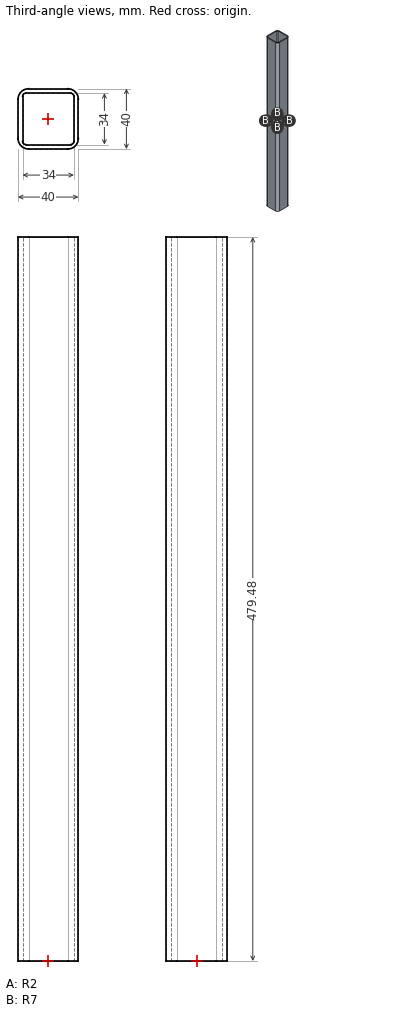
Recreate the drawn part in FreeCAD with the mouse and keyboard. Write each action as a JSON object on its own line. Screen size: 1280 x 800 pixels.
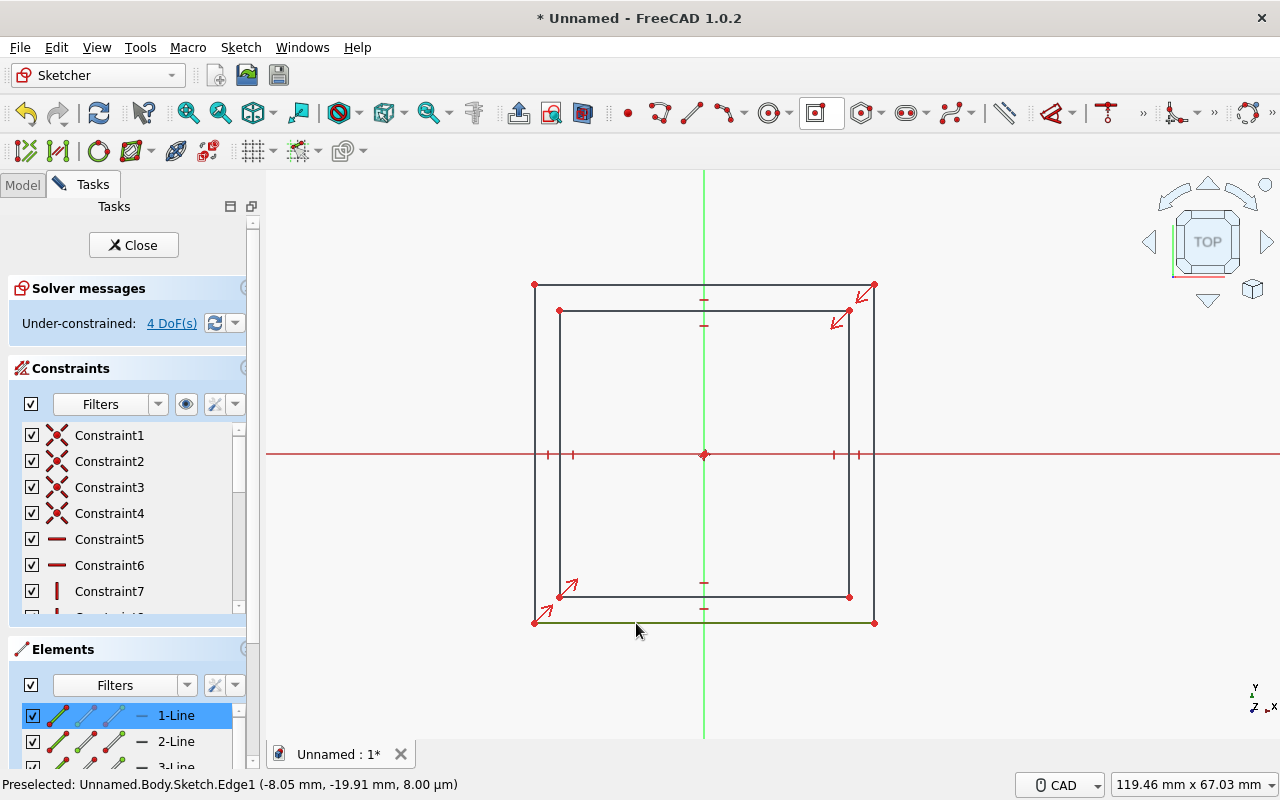
{"action": "left_click", "coordinate": [1074, 114]}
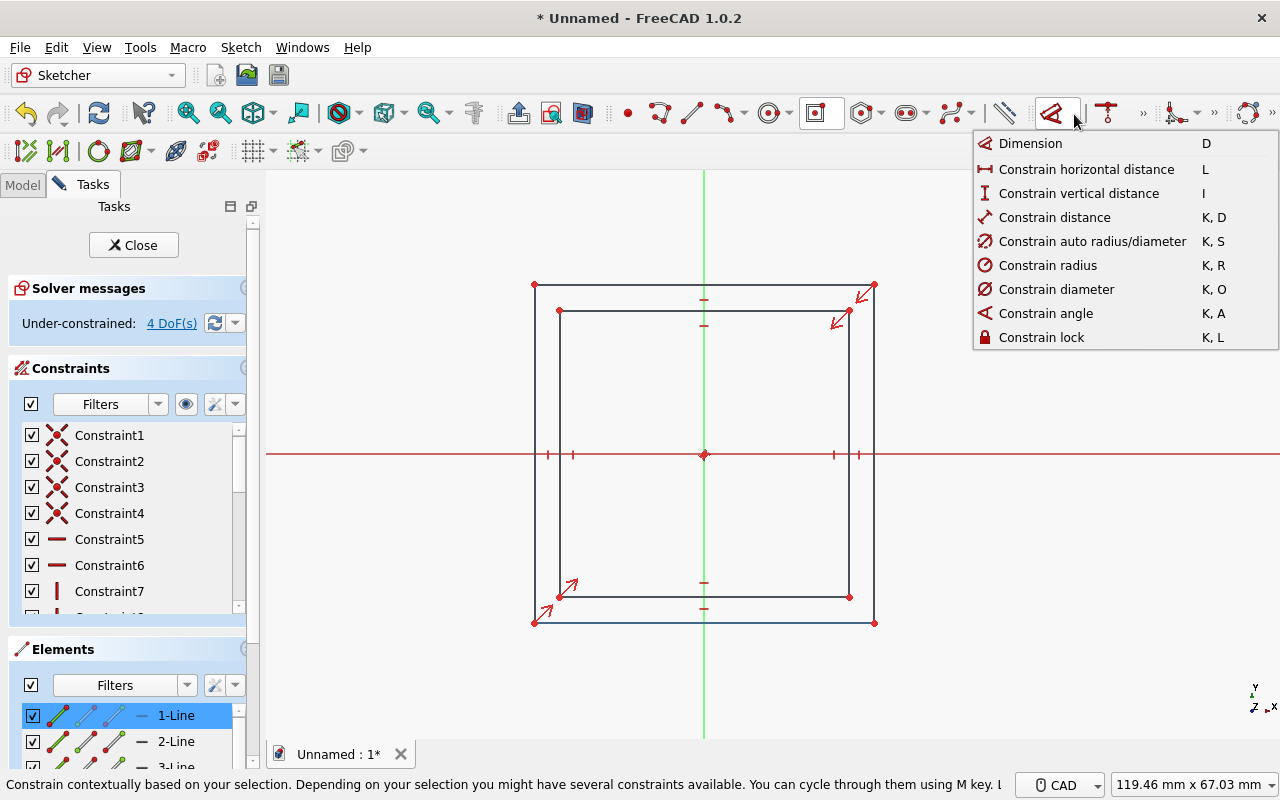
{"action": "left_click", "coordinate": [1126, 169]}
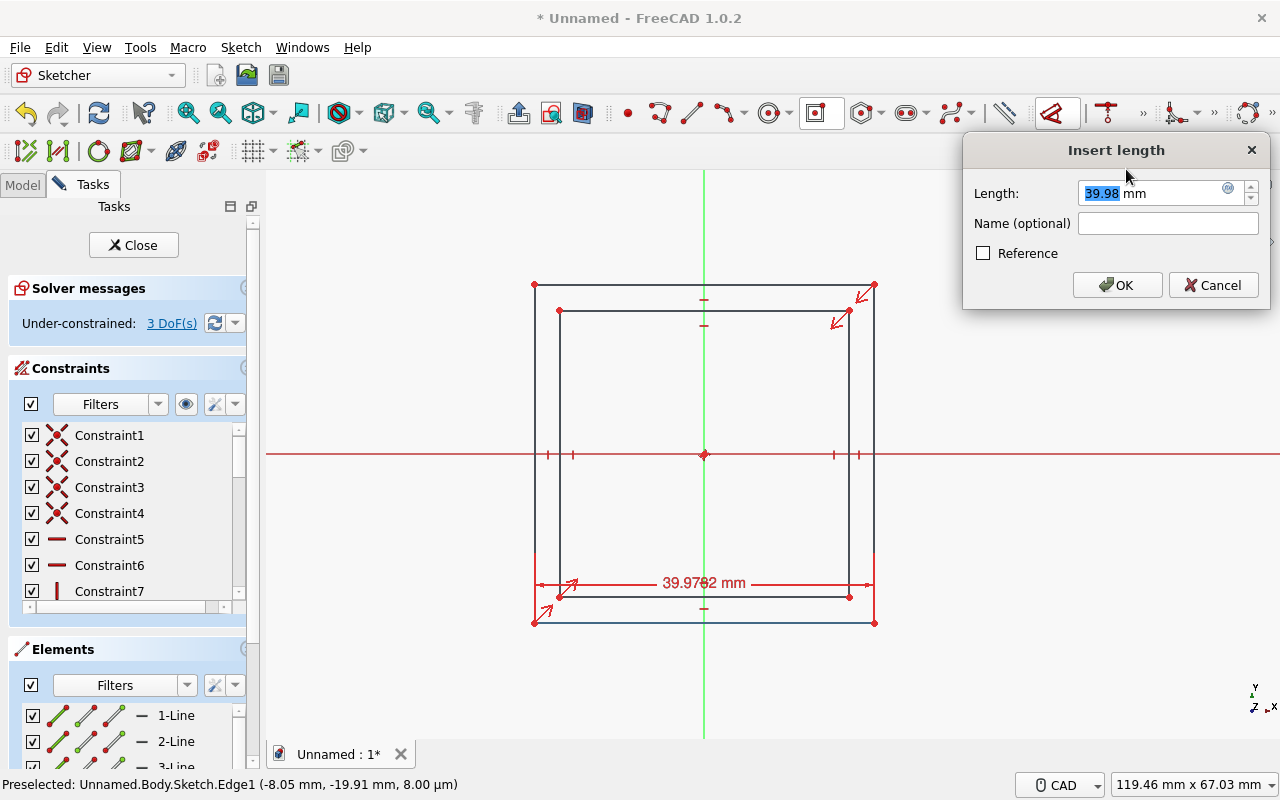
{"action": "type", "text": "40"}
{"action": "key", "text": "Return"}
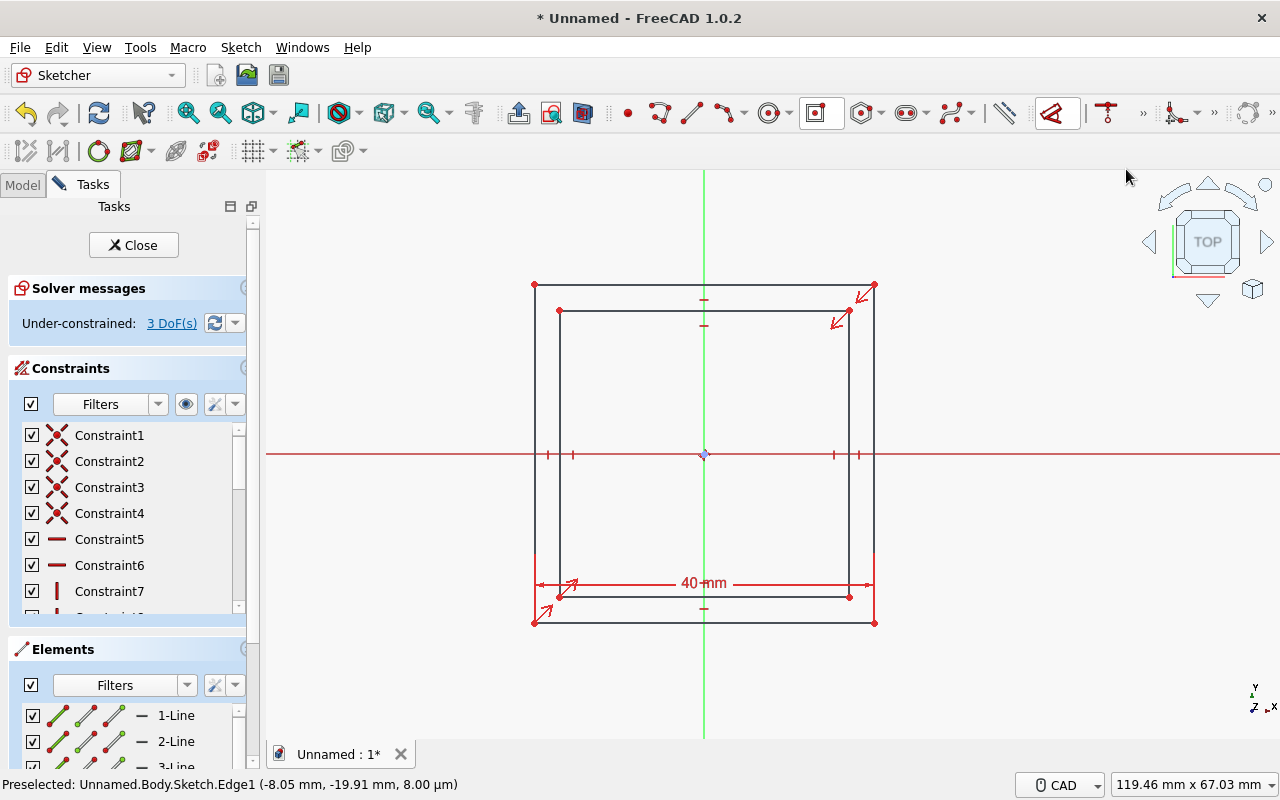
{"action": "left_click", "coordinate": [874, 522]}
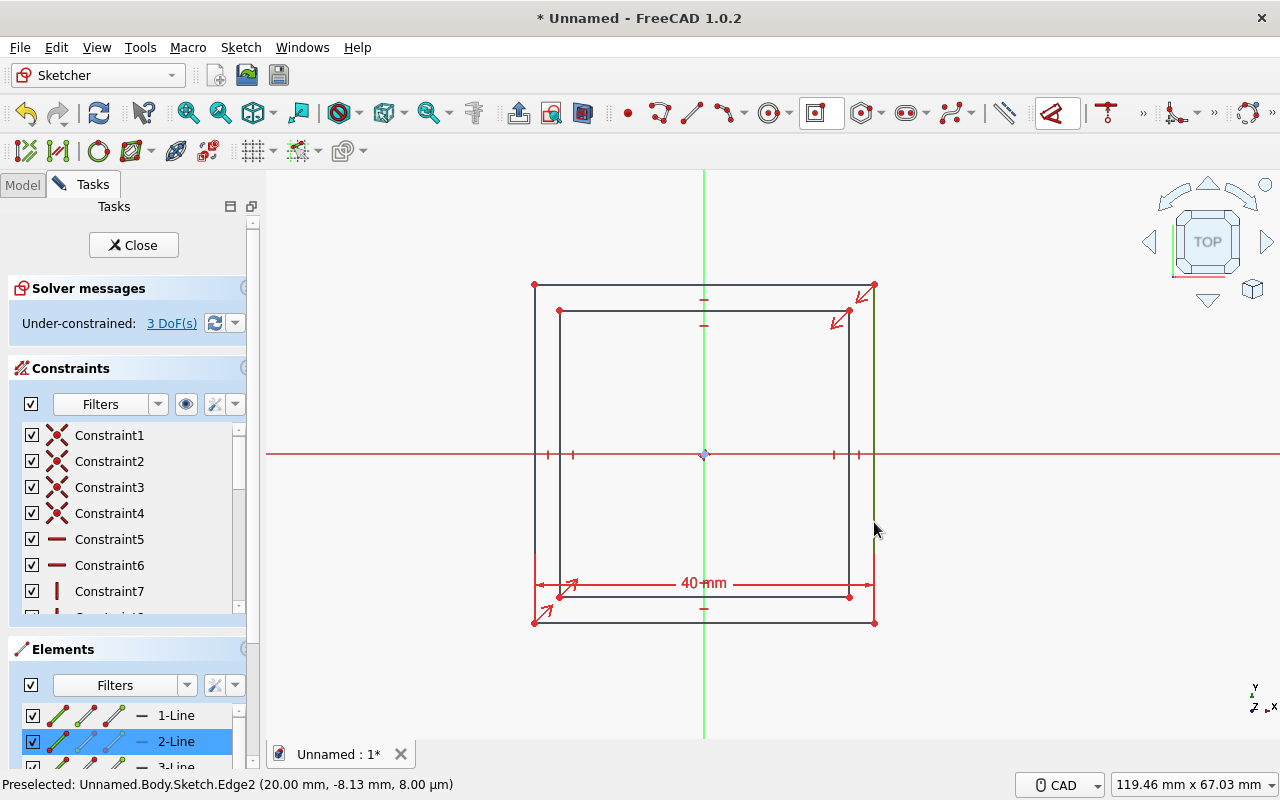
{"action": "key", "text": "i"}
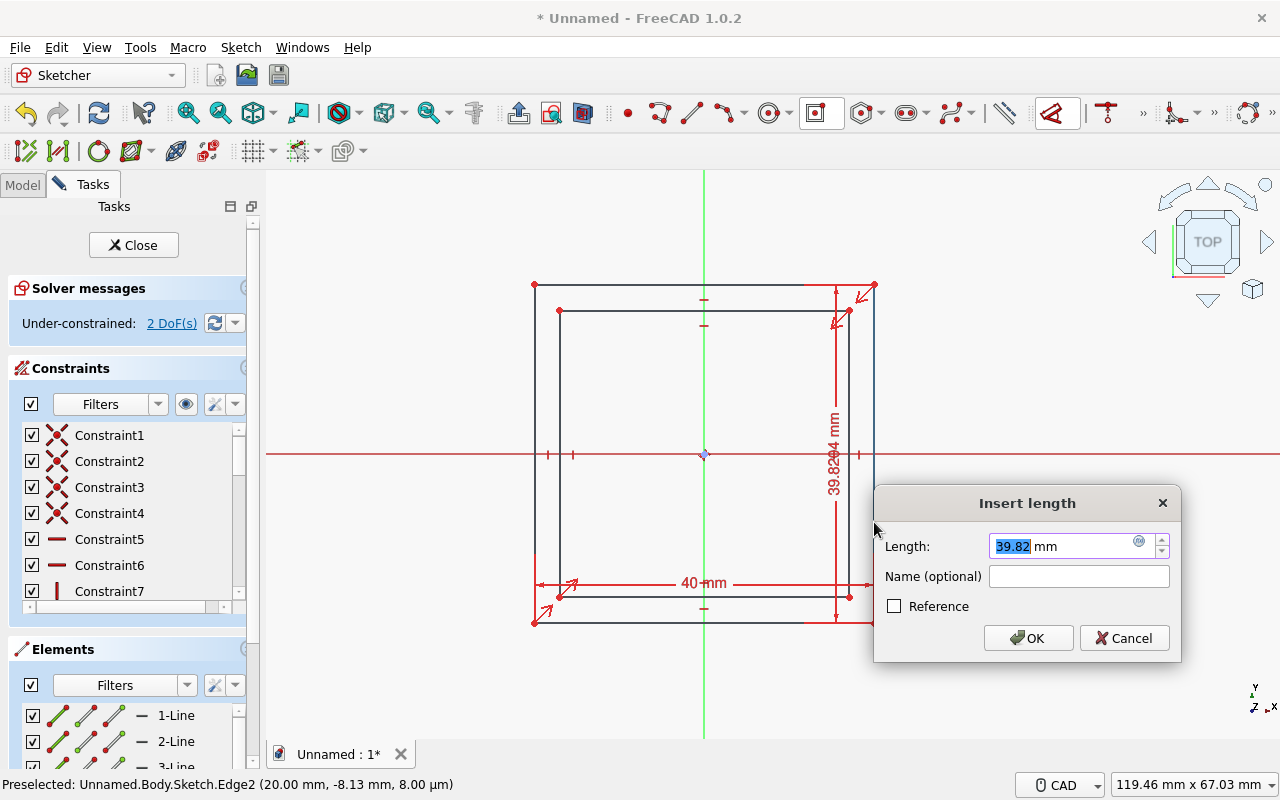
{"action": "type", "text": "40"}
{"action": "key", "text": "Return"}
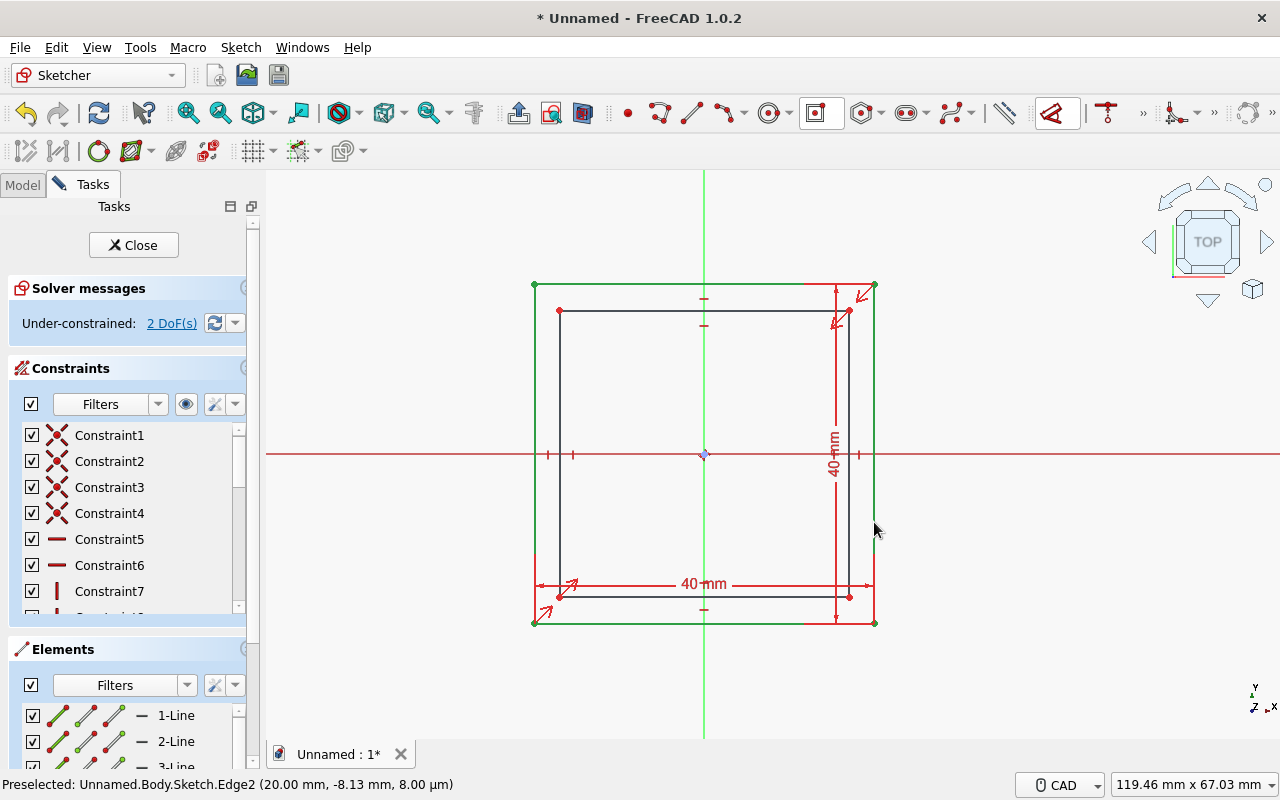
{"action": "left_click", "coordinate": [646, 597]}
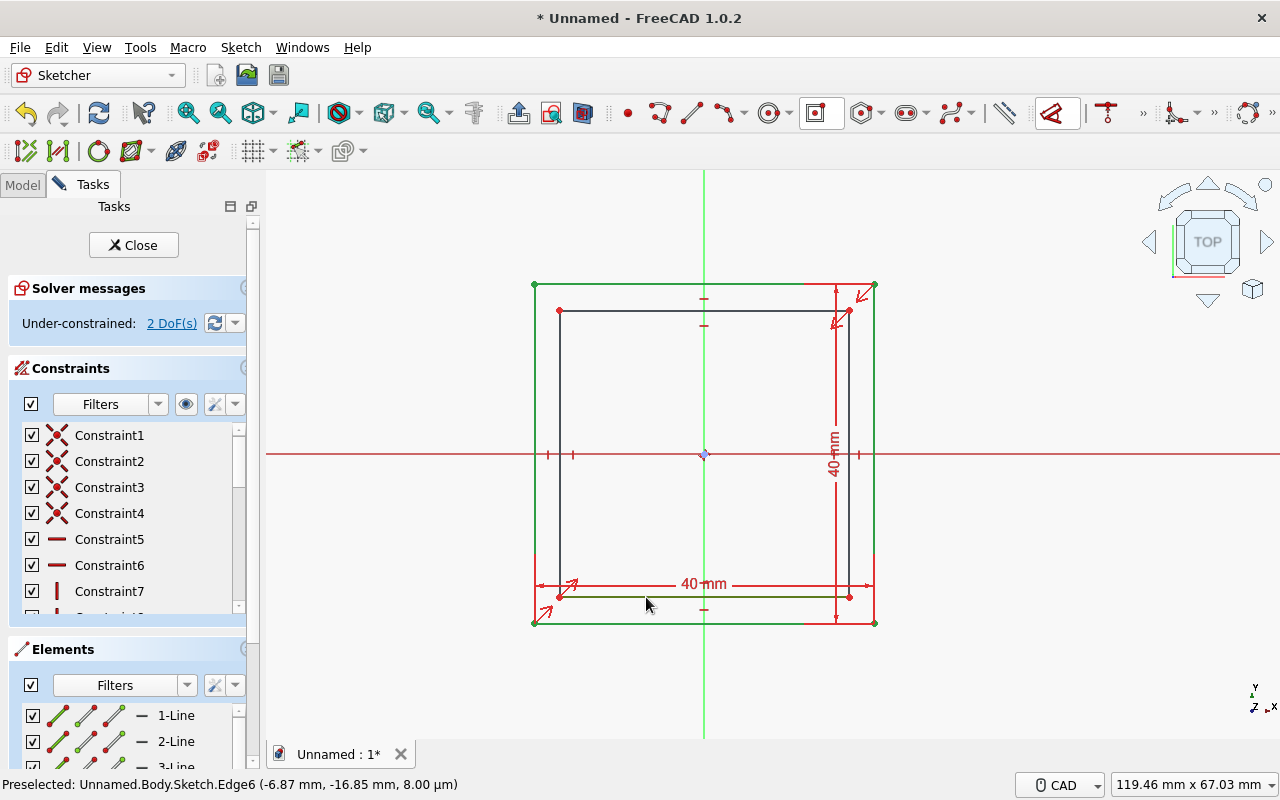
{"action": "key", "text": "l"}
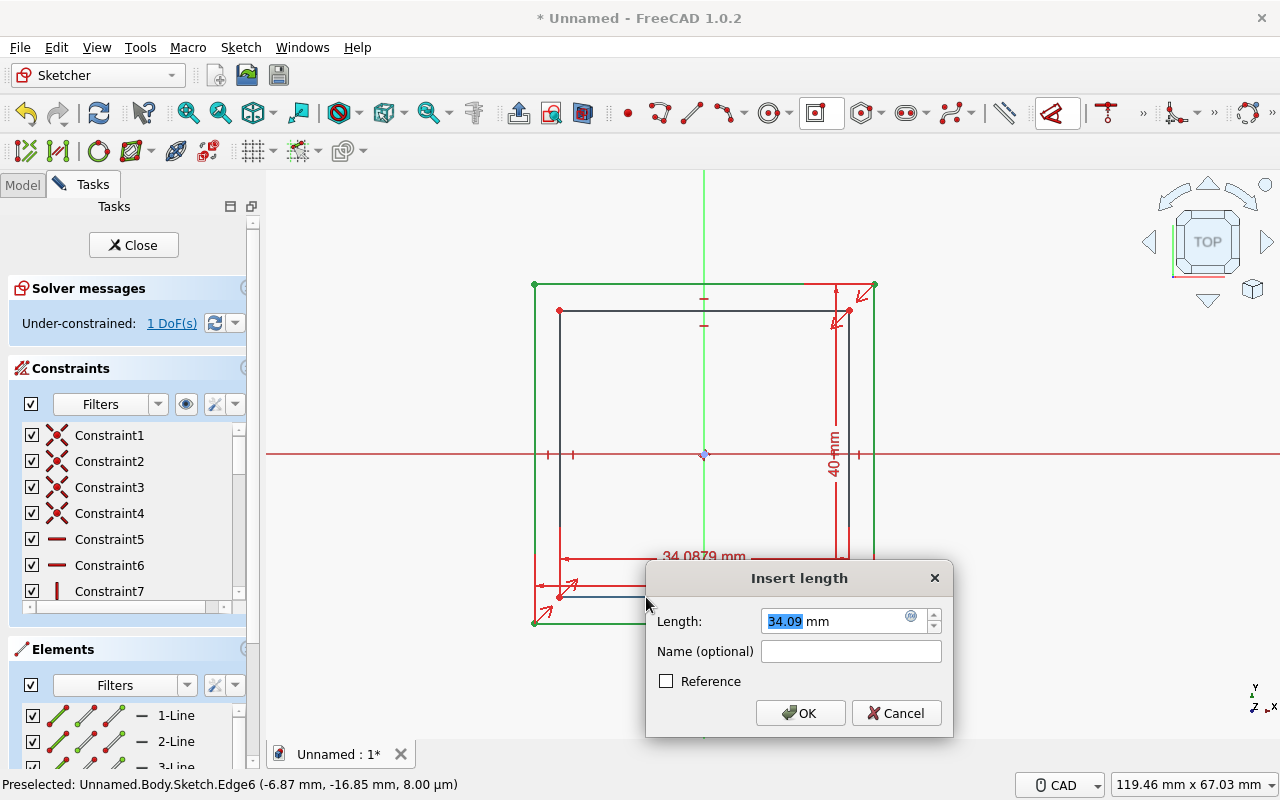
{"action": "type", "text": "34"}
{"action": "key", "text": "Return"}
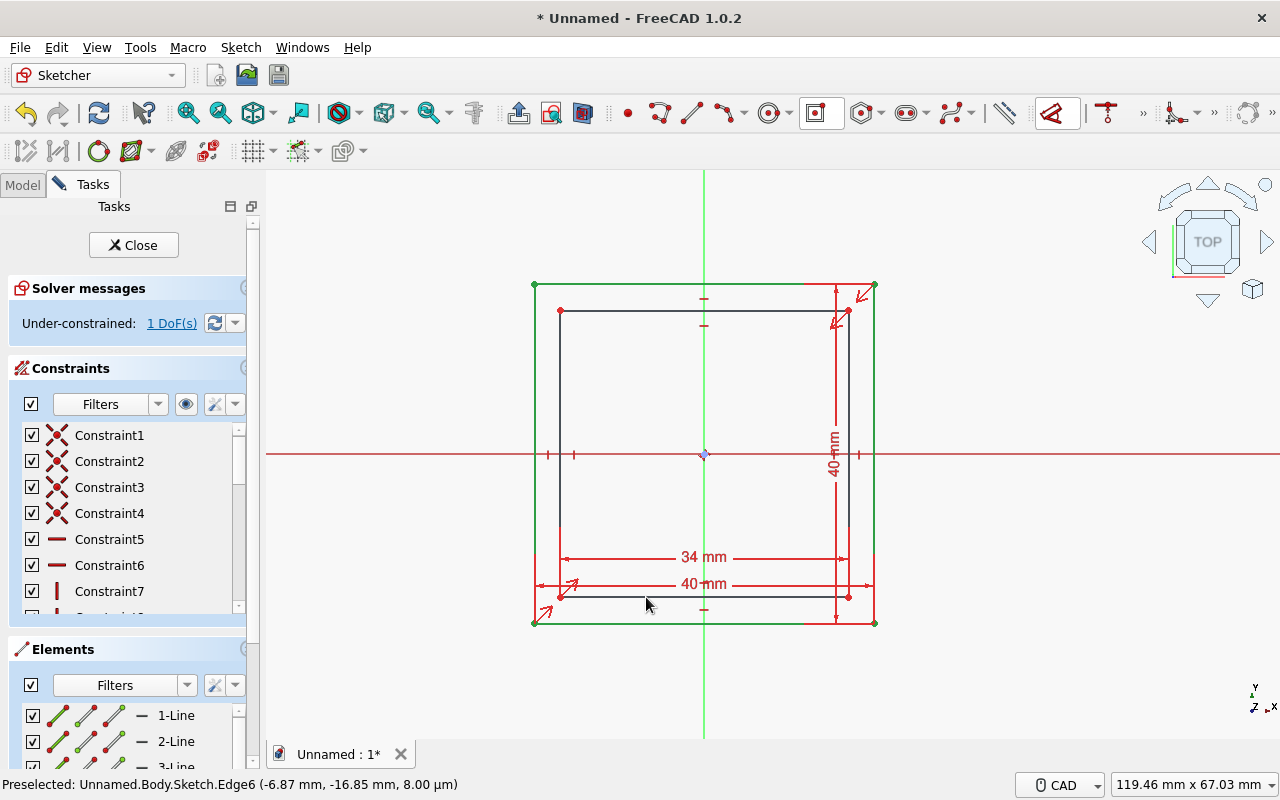
{"action": "left_click", "coordinate": [849, 511]}